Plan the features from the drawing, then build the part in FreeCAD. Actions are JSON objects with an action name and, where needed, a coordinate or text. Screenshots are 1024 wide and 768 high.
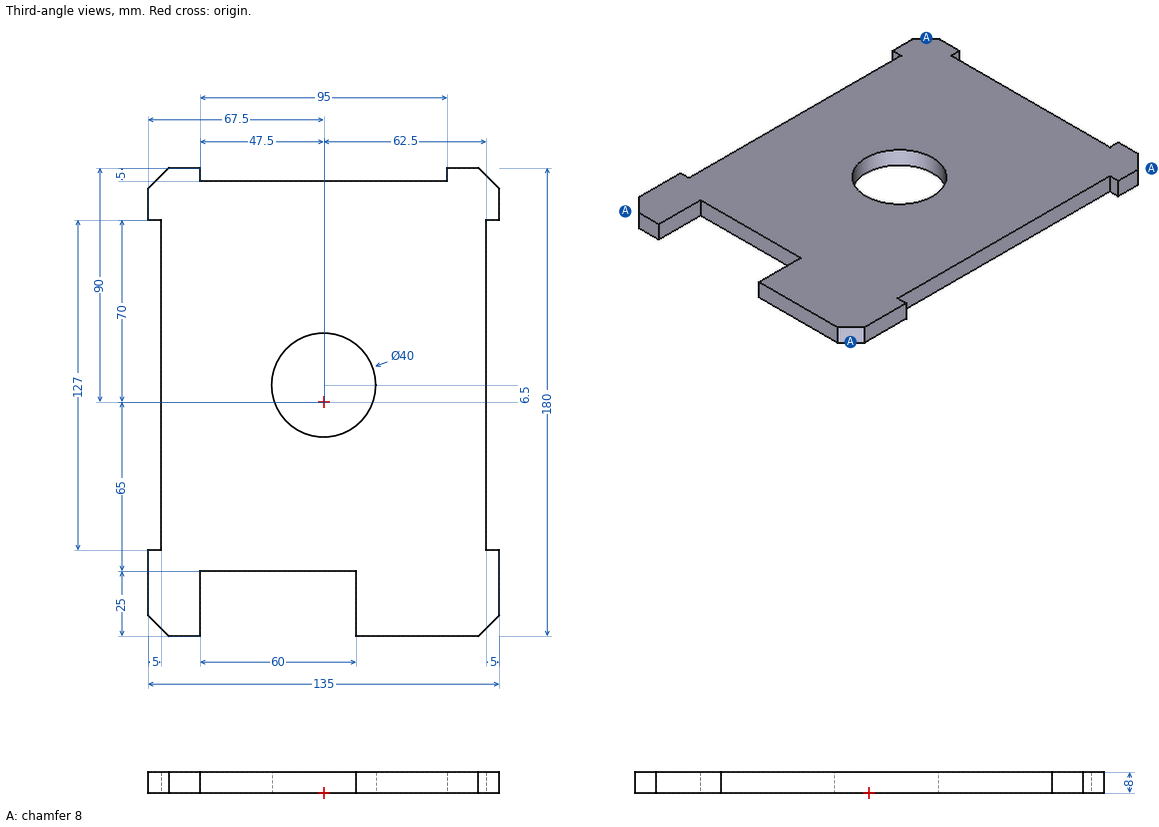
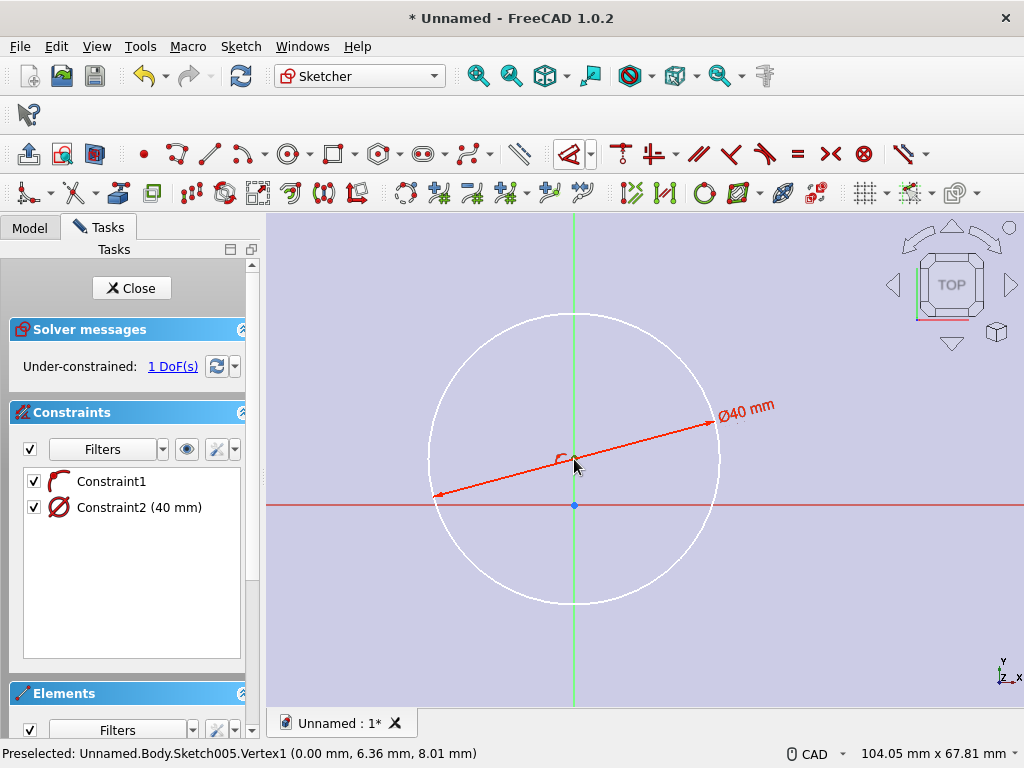
{"action": "key", "text": "i"}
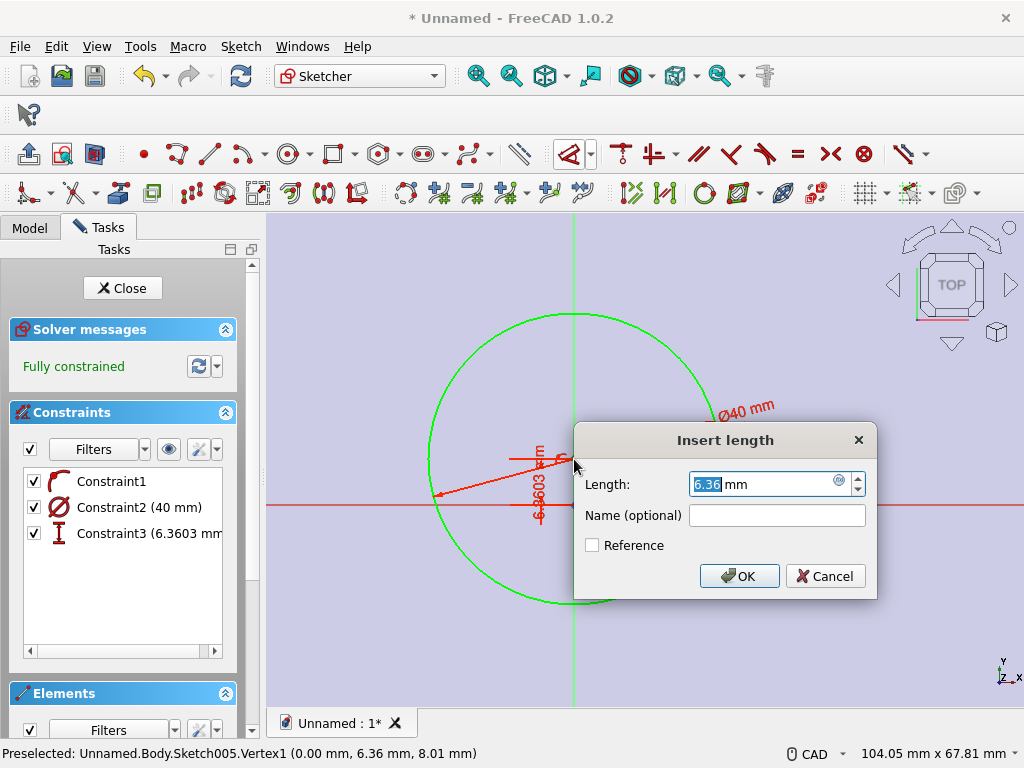
{"action": "type", "text": "6.5"}
{"action": "key", "text": "Return"}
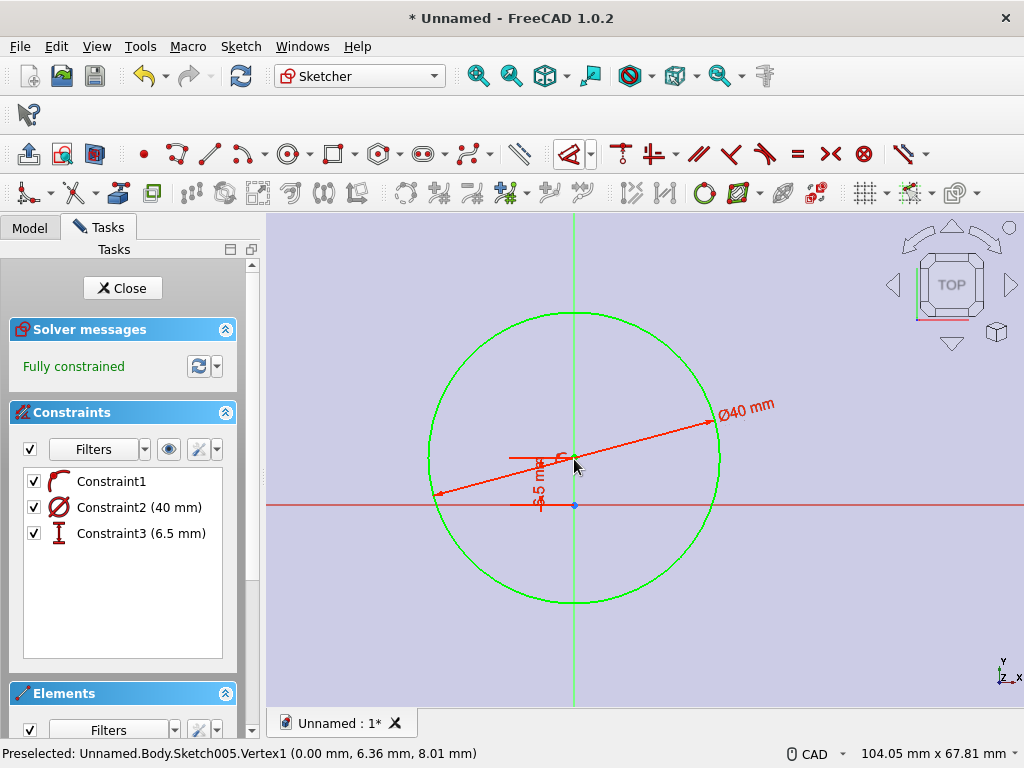
{"action": "left_click", "coordinate": [123, 288]}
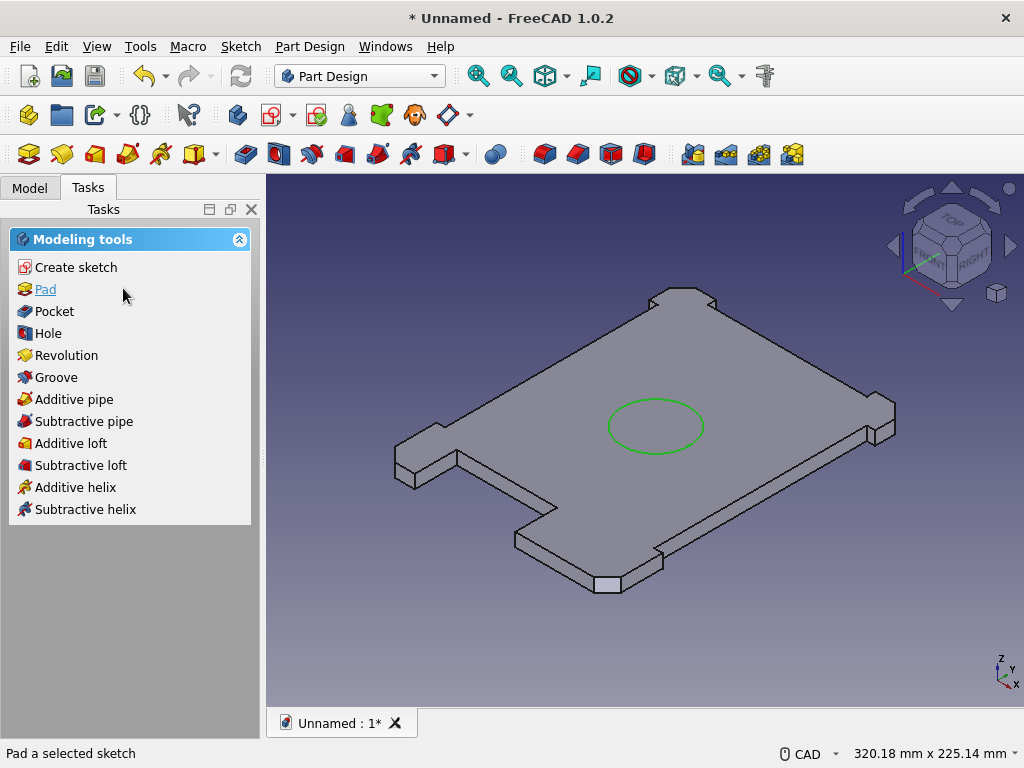
{"action": "left_click", "coordinate": [246, 154]}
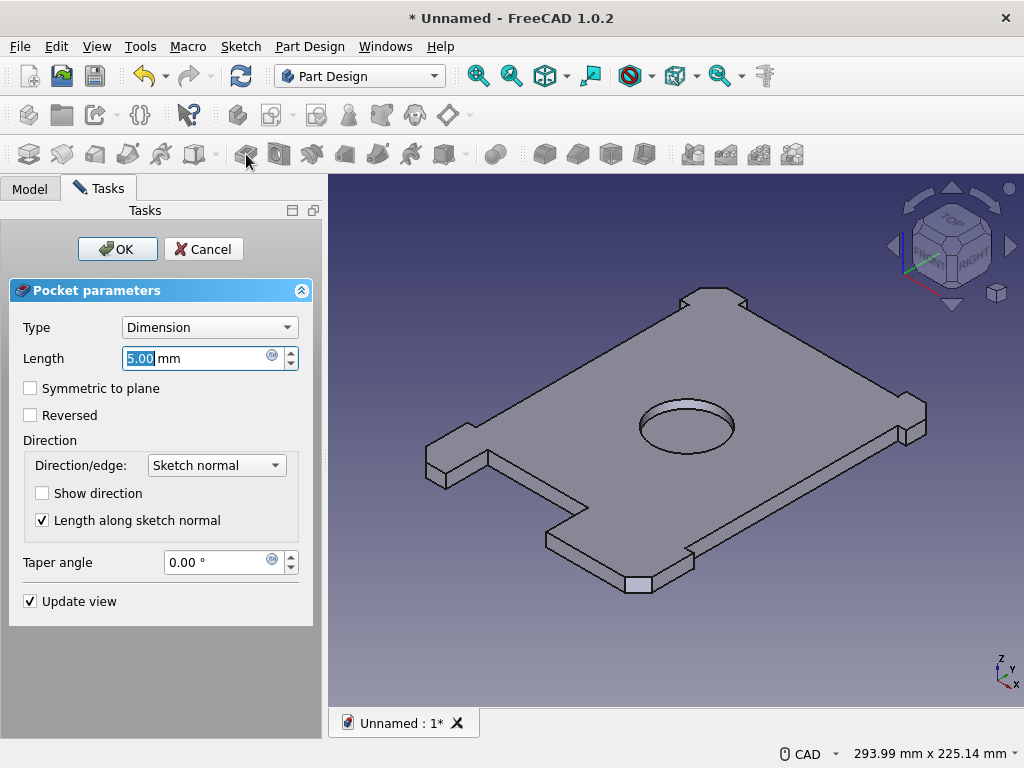
{"action": "left_click", "coordinate": [210, 328]}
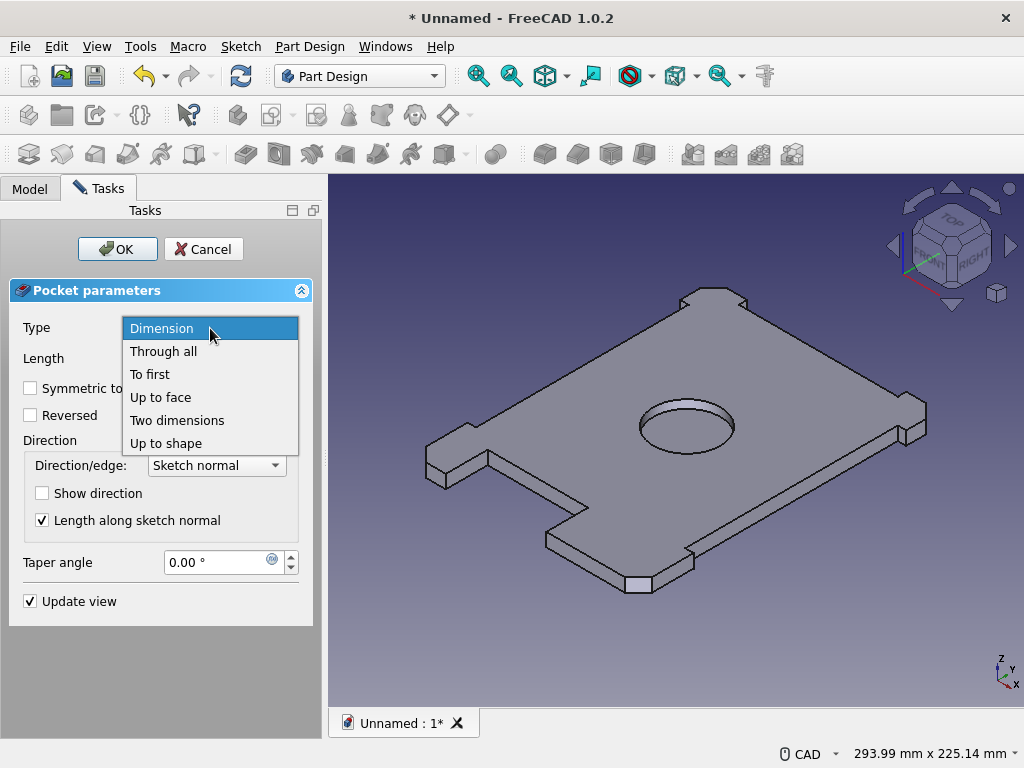
{"action": "left_click", "coordinate": [208, 374]}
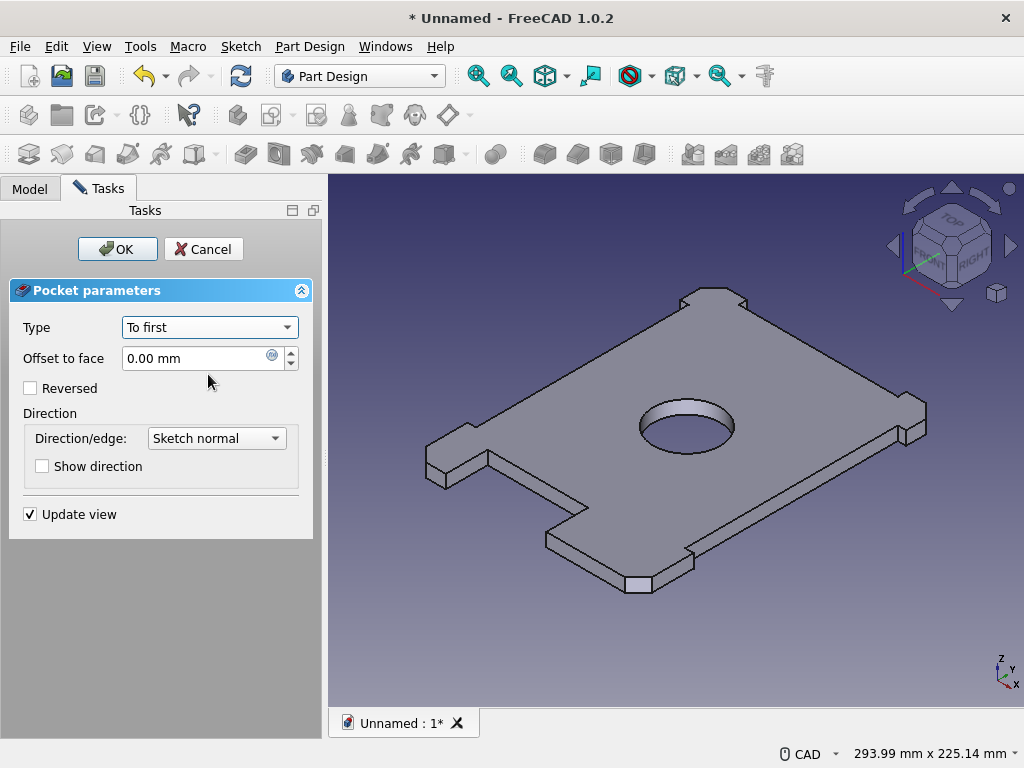
{"action": "left_click", "coordinate": [118, 249]}